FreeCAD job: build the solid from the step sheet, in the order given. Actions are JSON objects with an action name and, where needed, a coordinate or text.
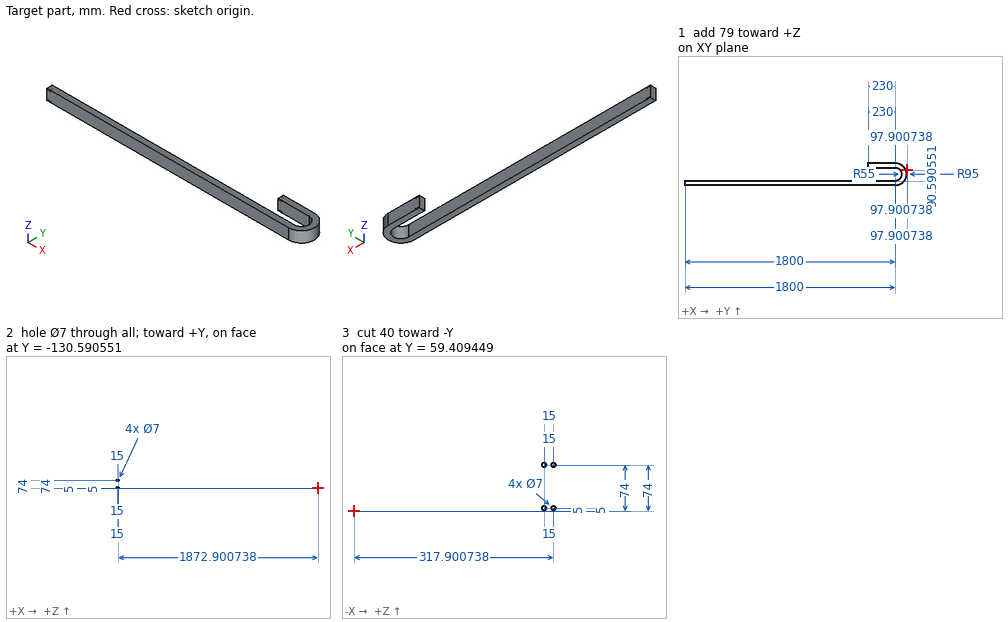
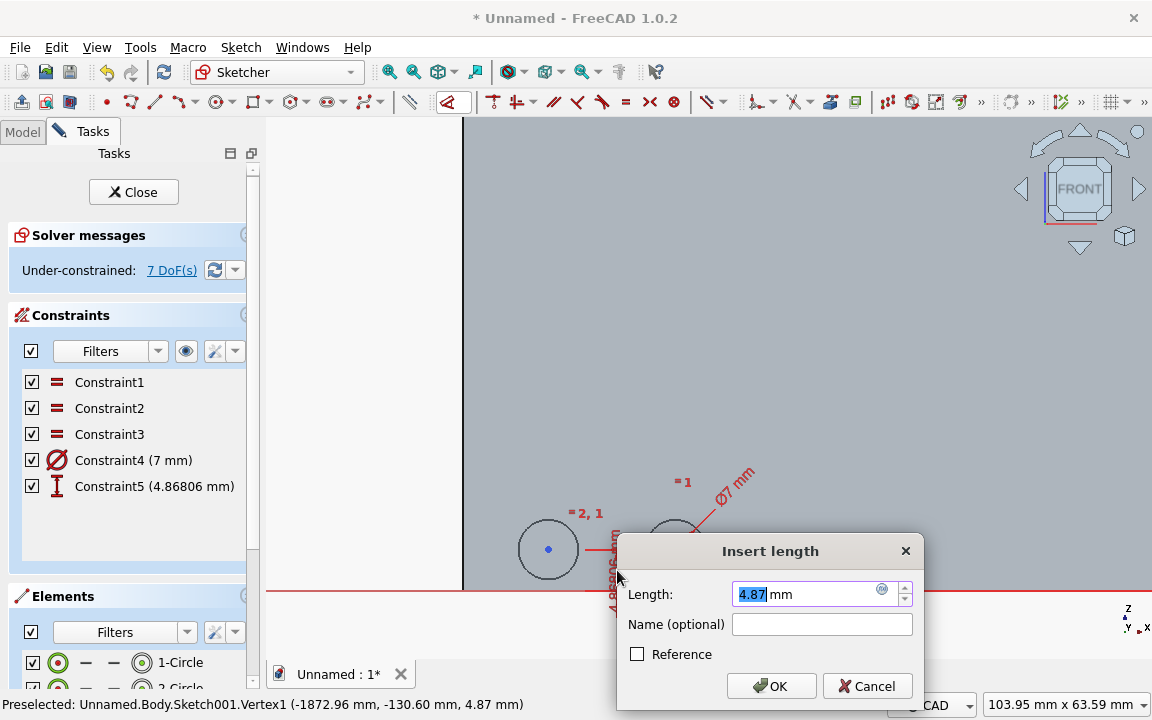
{"action": "type", "text": "5"}
{"action": "key", "text": "Return"}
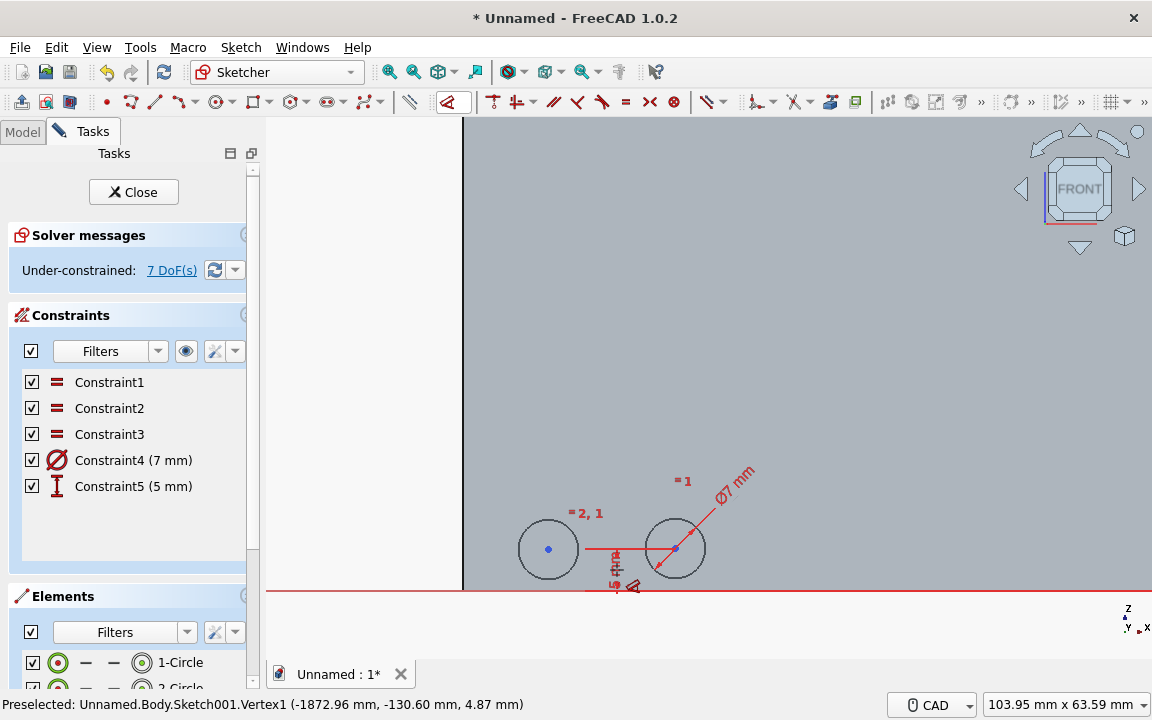
{"action": "left_click", "coordinate": [548, 550]}
{"action": "left_click", "coordinate": [490, 570]}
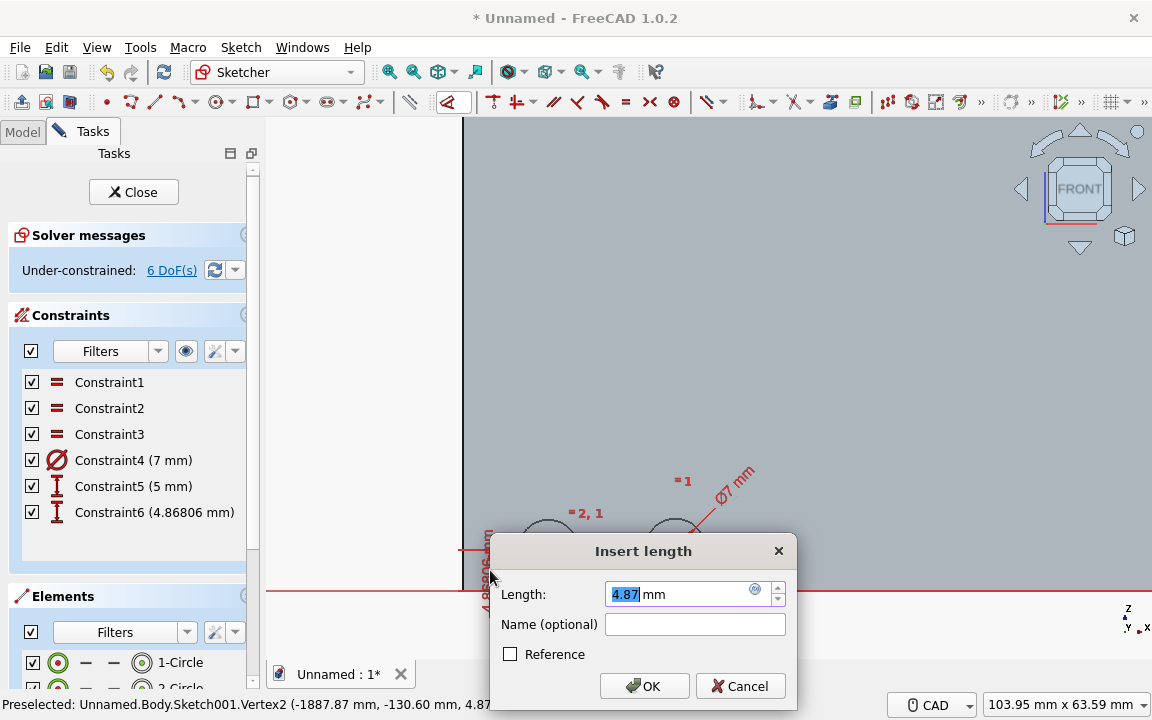
{"action": "type", "text": "5"}
{"action": "key", "text": "Return"}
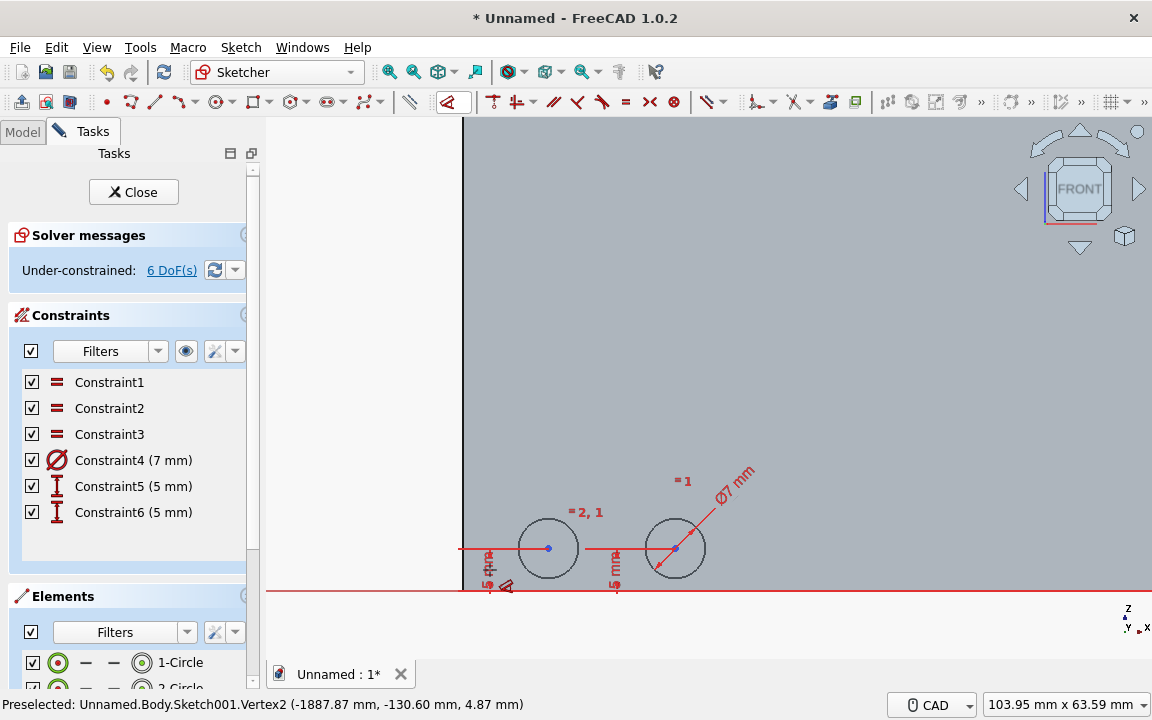
{"action": "scroll", "coordinate": [675, 550], "scroll_direction": "down", "scroll_amount": 3}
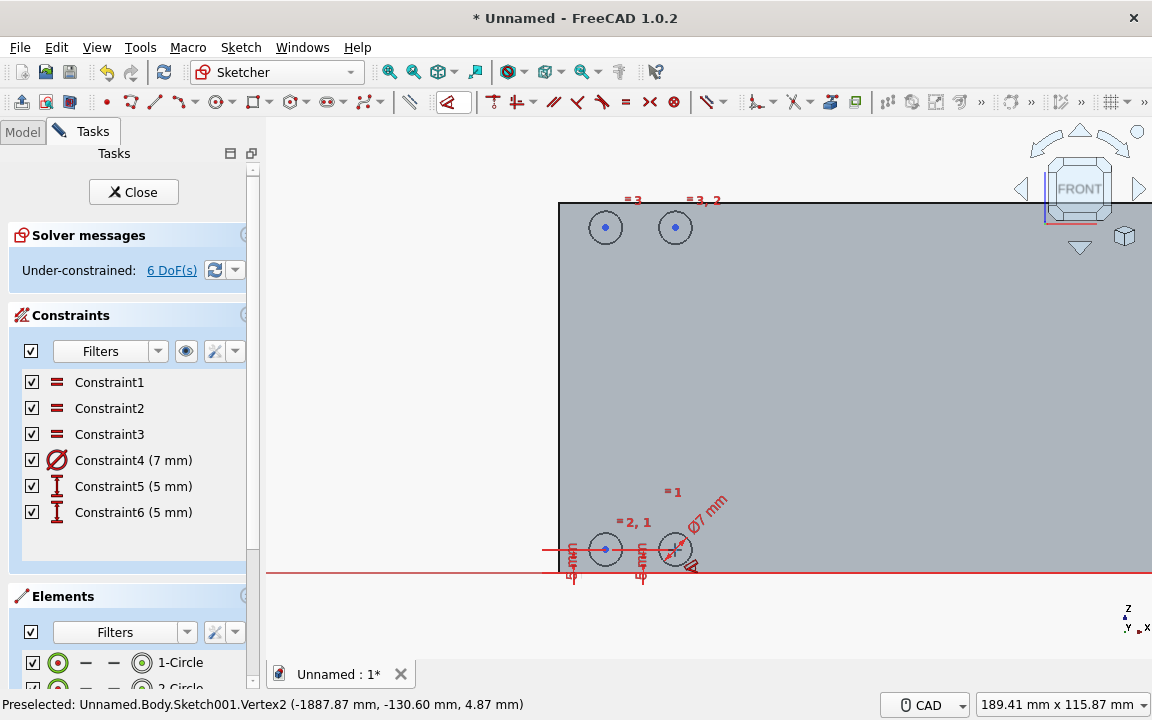
{"action": "left_click", "coordinate": [675, 228]}
{"action": "left_click", "coordinate": [641, 400]}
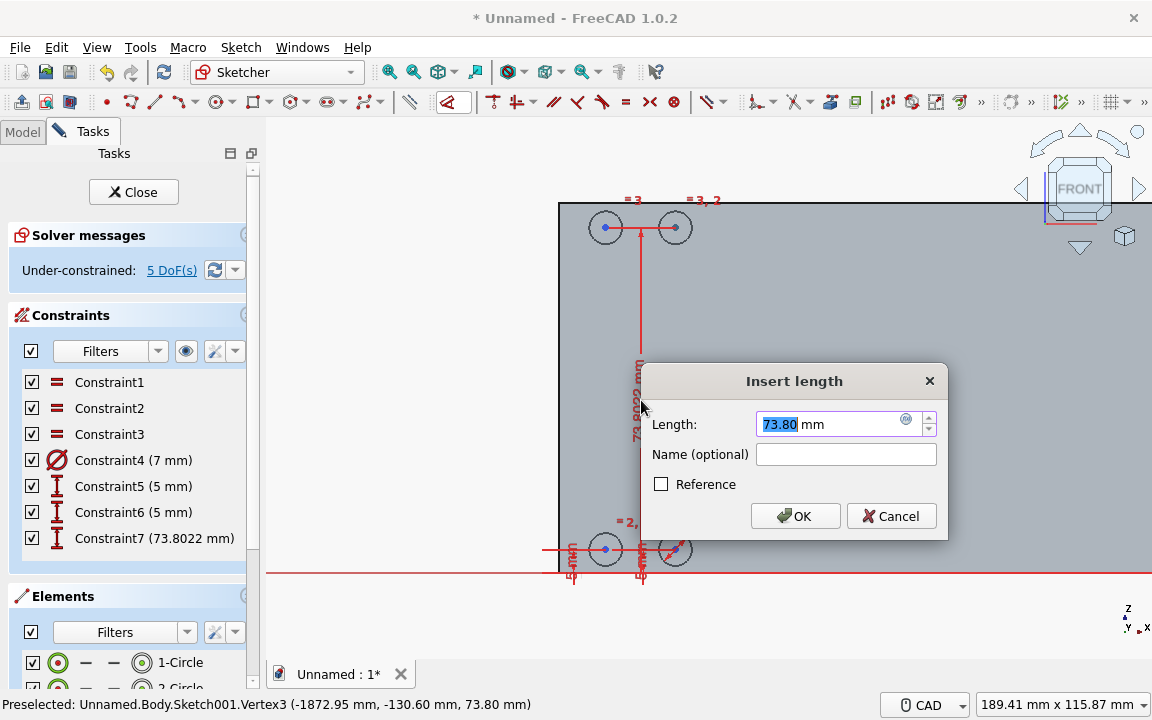
{"action": "type", "text": "74"}
{"action": "key", "text": "Return"}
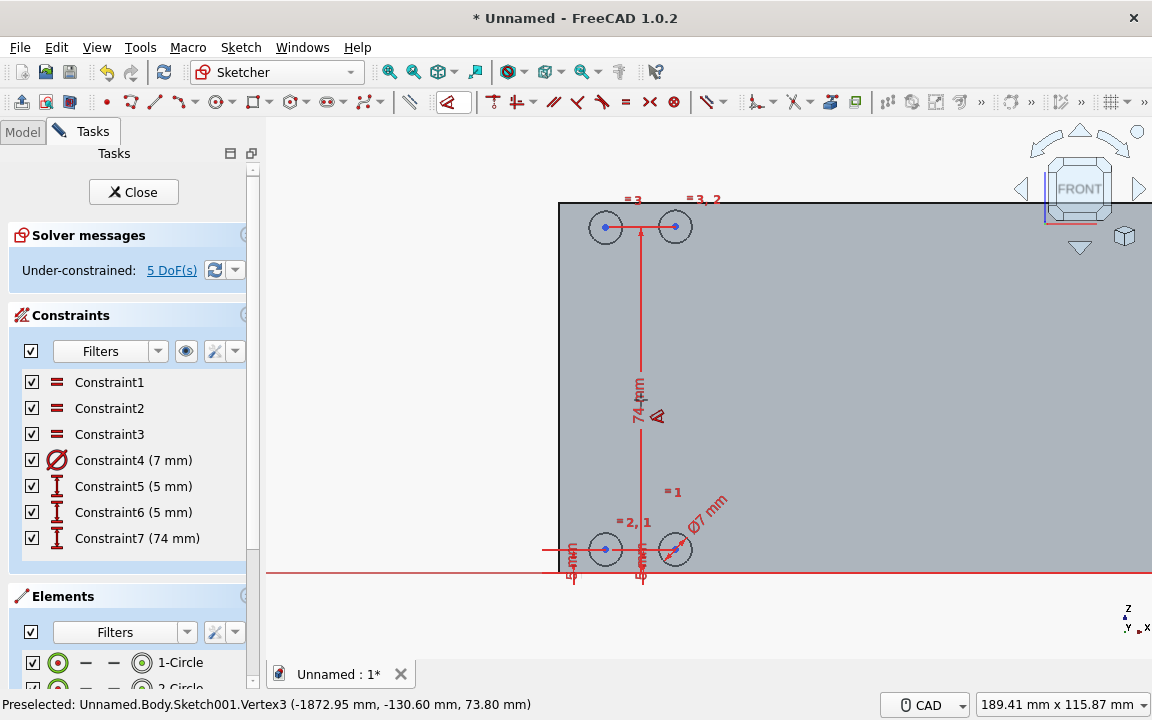
{"action": "left_click", "coordinate": [606, 228]}
{"action": "left_click", "coordinate": [572, 321]}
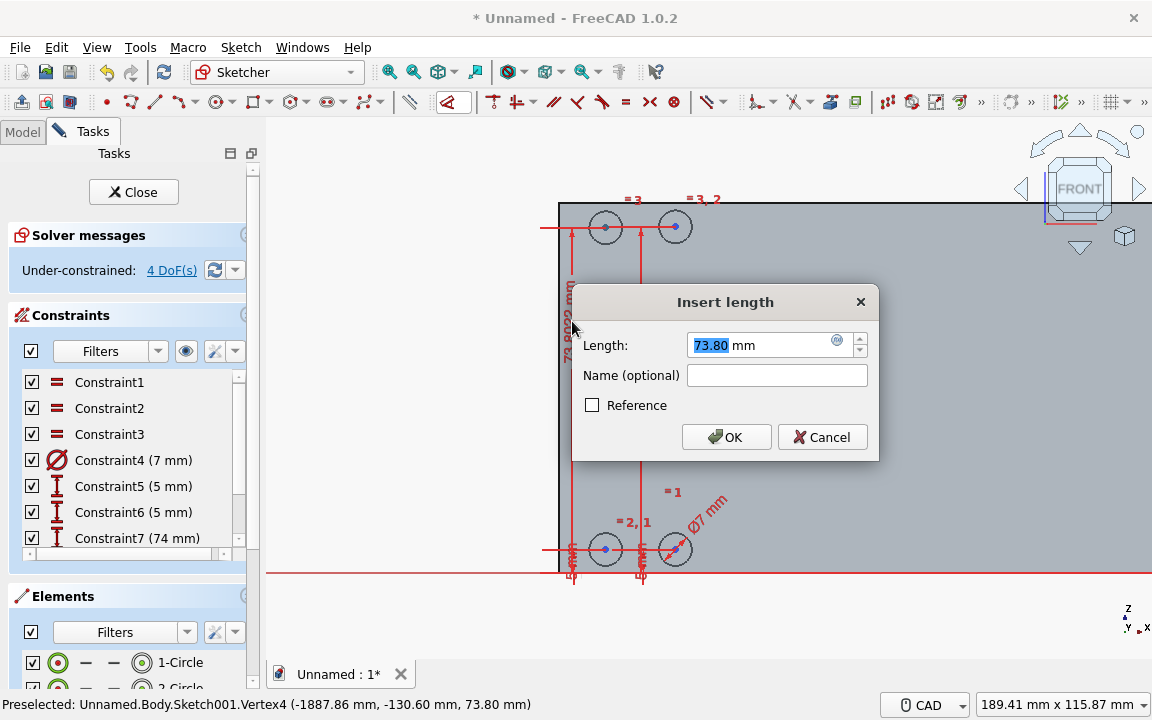
{"action": "type", "text": "74"}
{"action": "key", "text": "Return"}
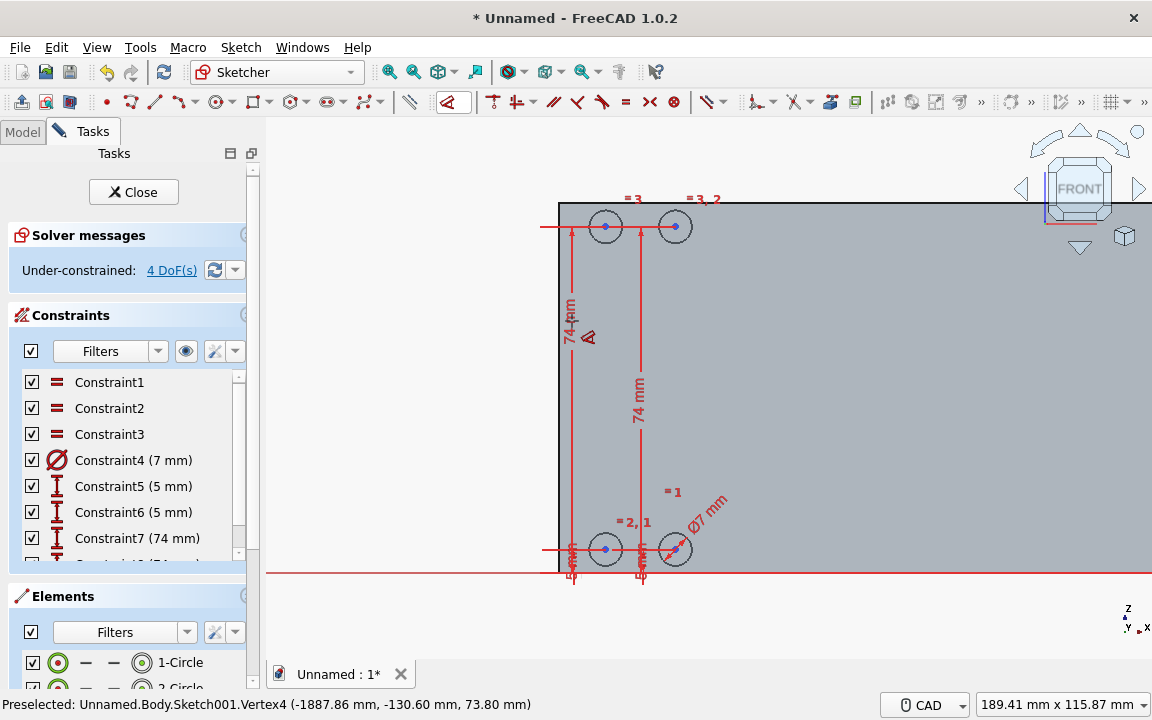
{"action": "left_click", "coordinate": [675, 550]}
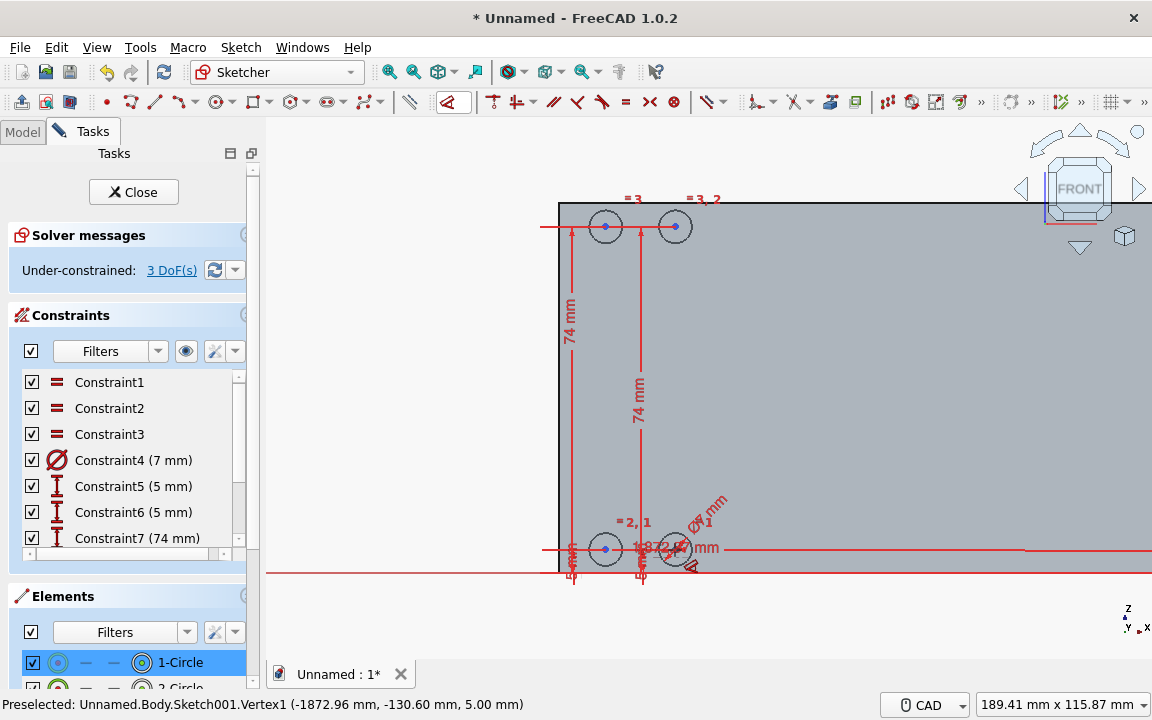
{"action": "left_click", "coordinate": [606, 550]}
{"action": "left_click", "coordinate": [625, 516]}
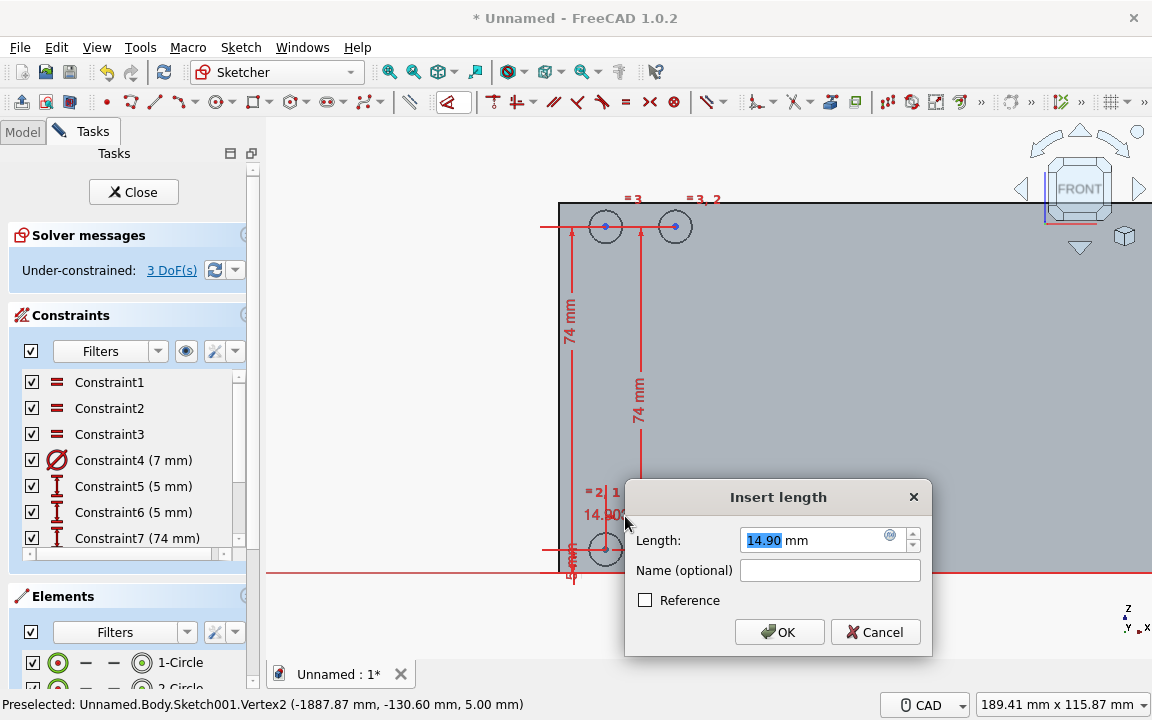
{"action": "type", "text": "15"}
{"action": "key", "text": "Return"}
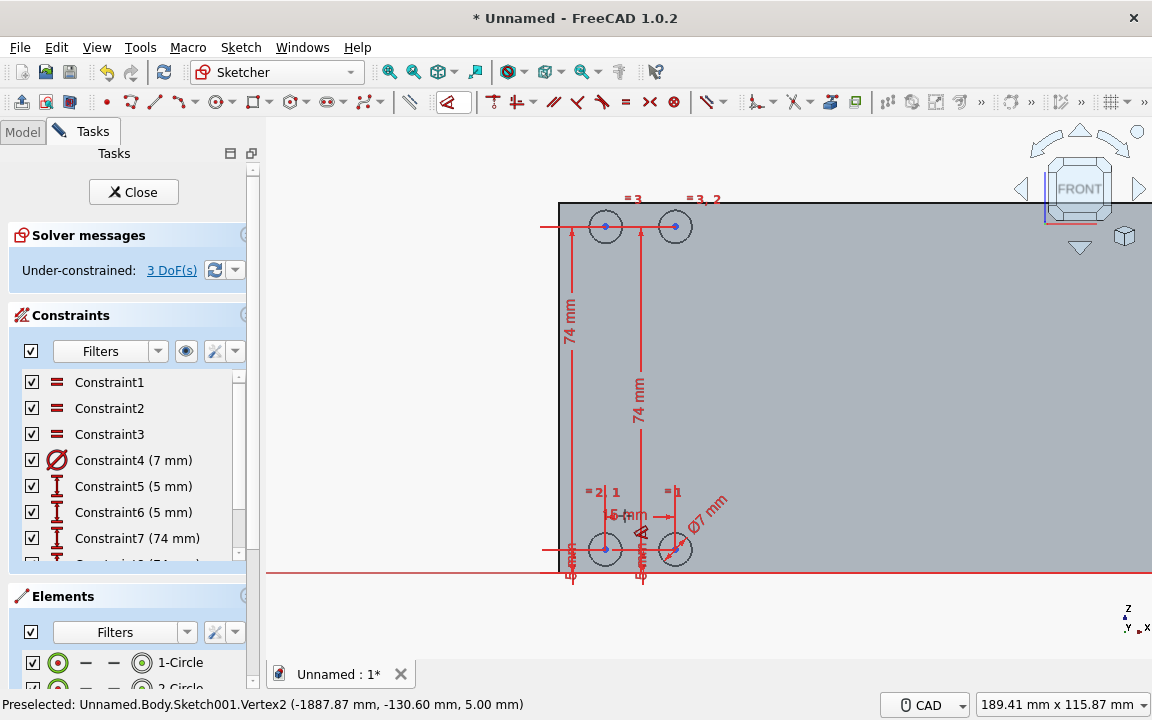
{"action": "left_click", "coordinate": [605, 550]}